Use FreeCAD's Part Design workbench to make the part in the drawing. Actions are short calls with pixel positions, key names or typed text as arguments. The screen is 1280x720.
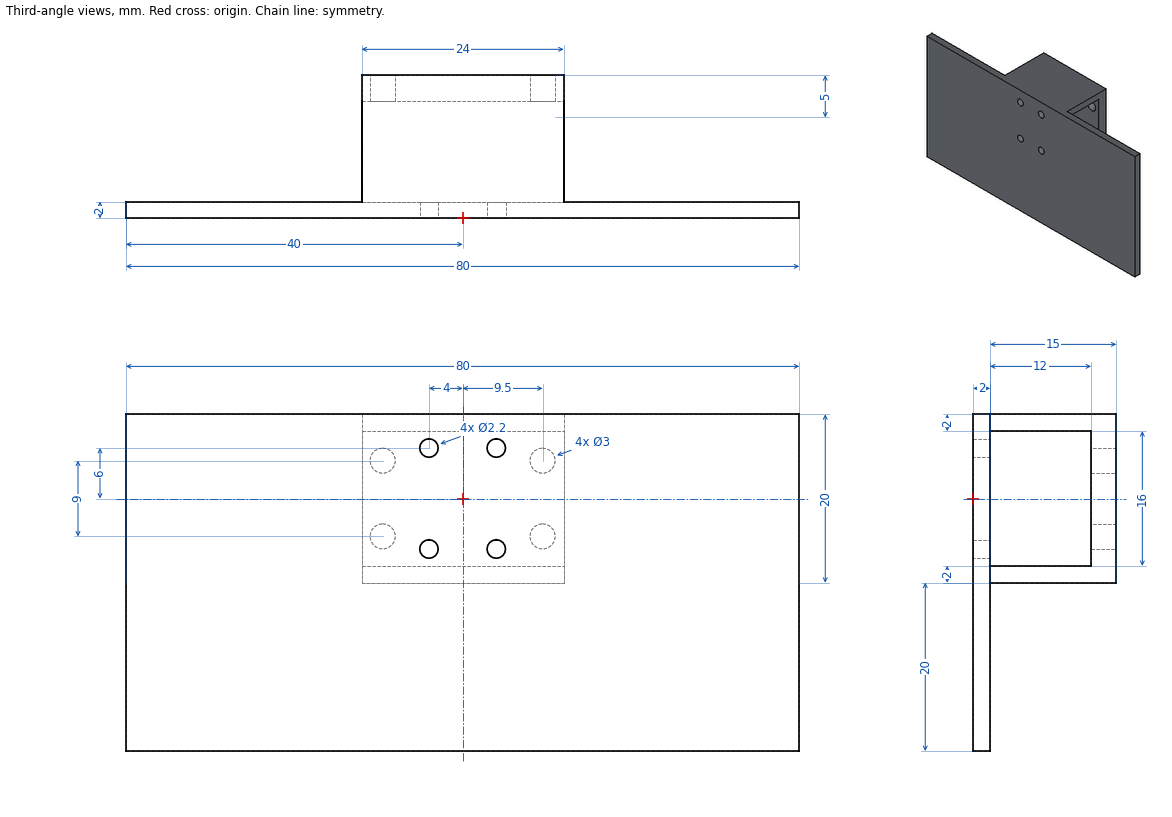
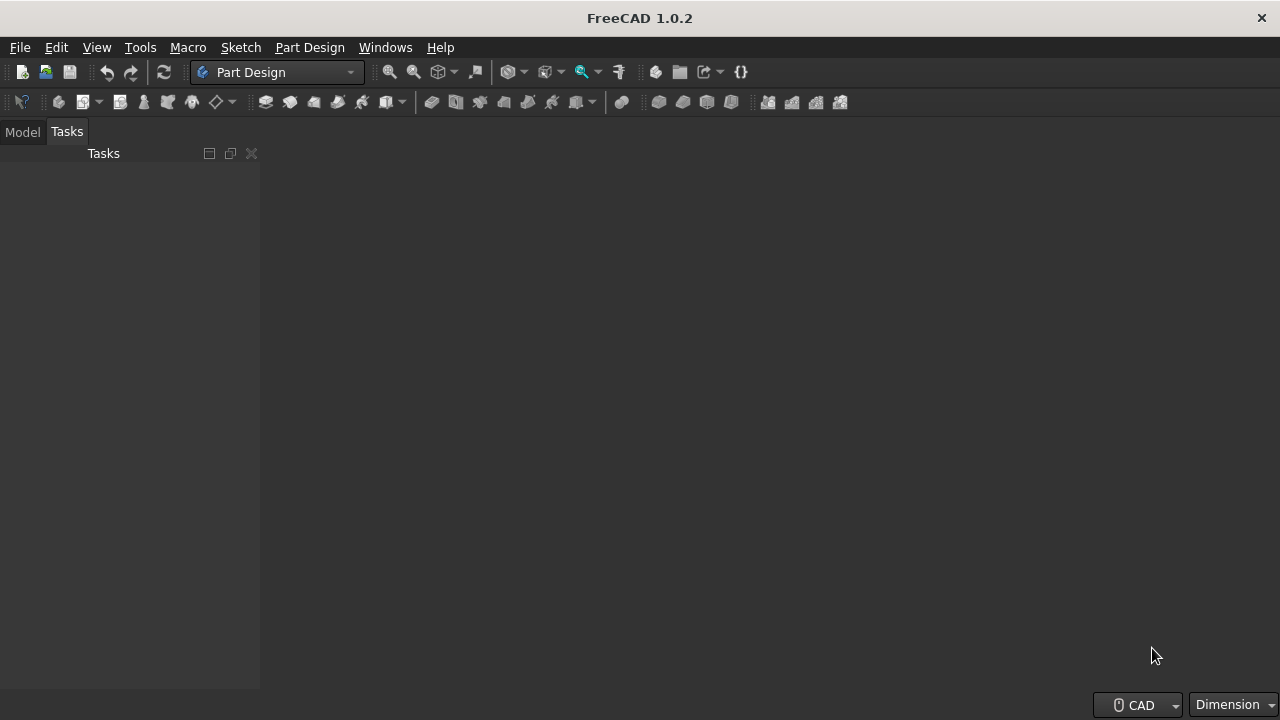
click(22, 72)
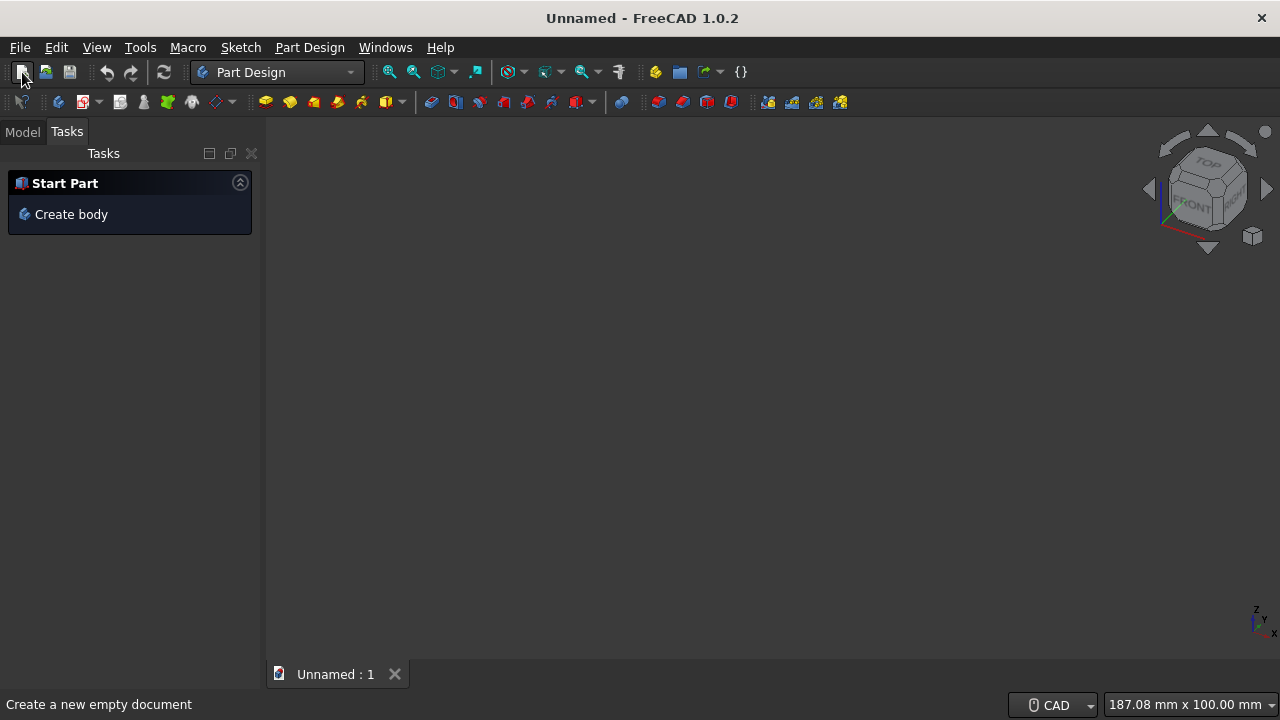
click(84, 102)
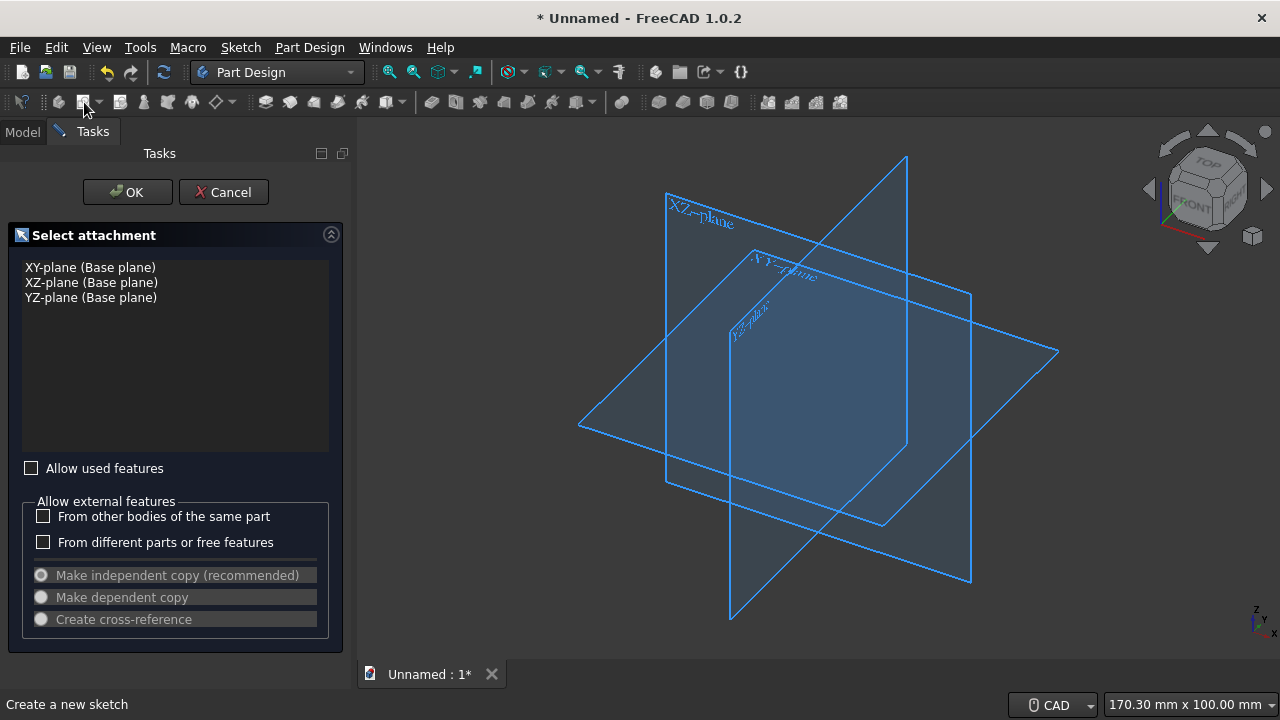
click(82, 282)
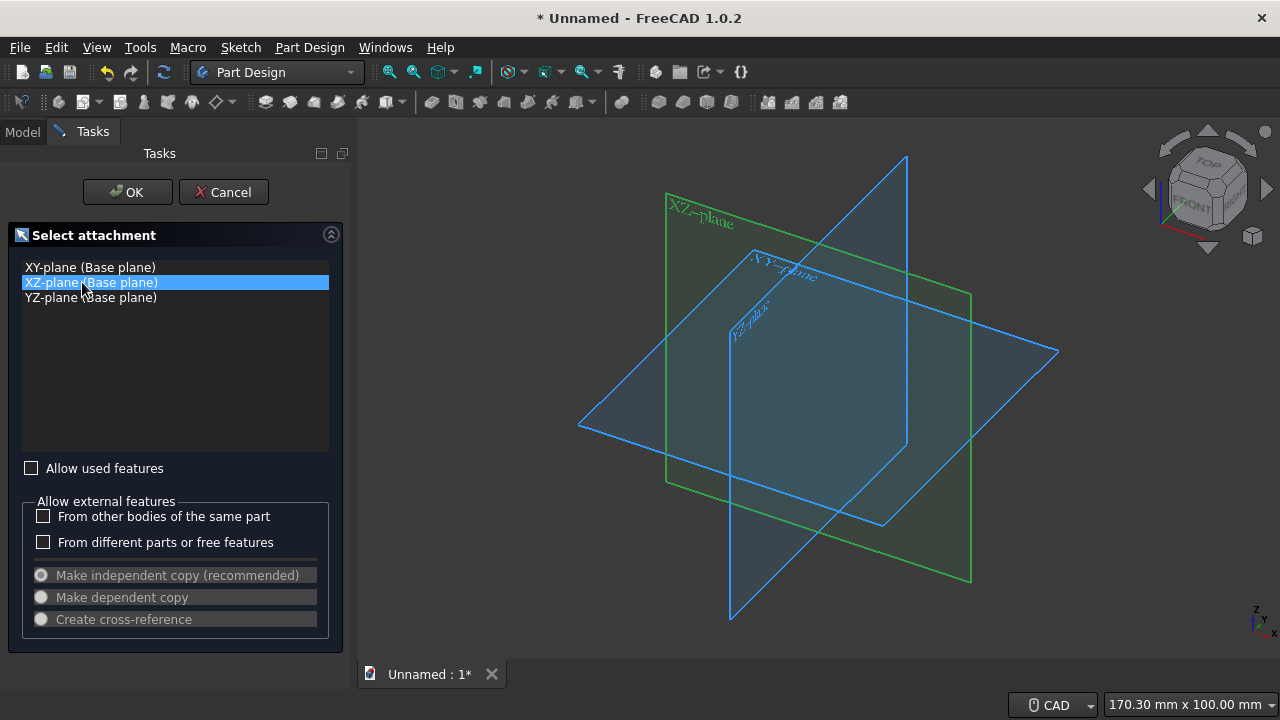
click(128, 192)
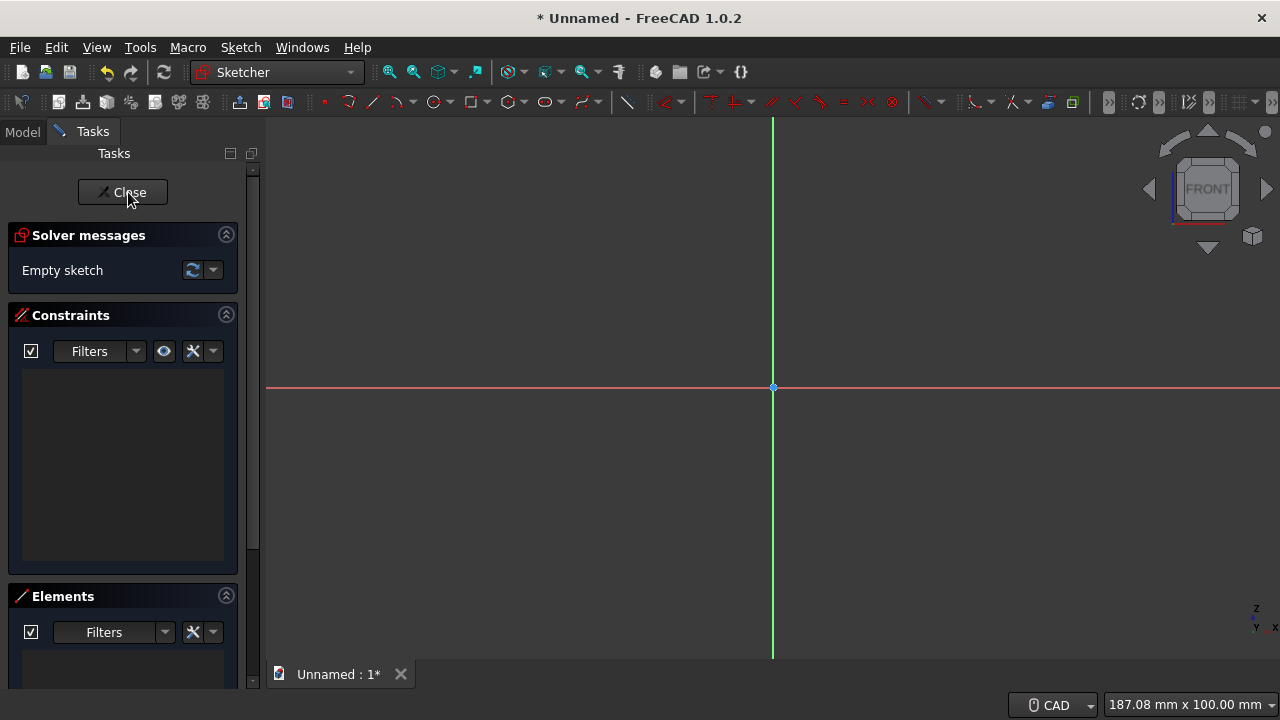
key(g)
key(v)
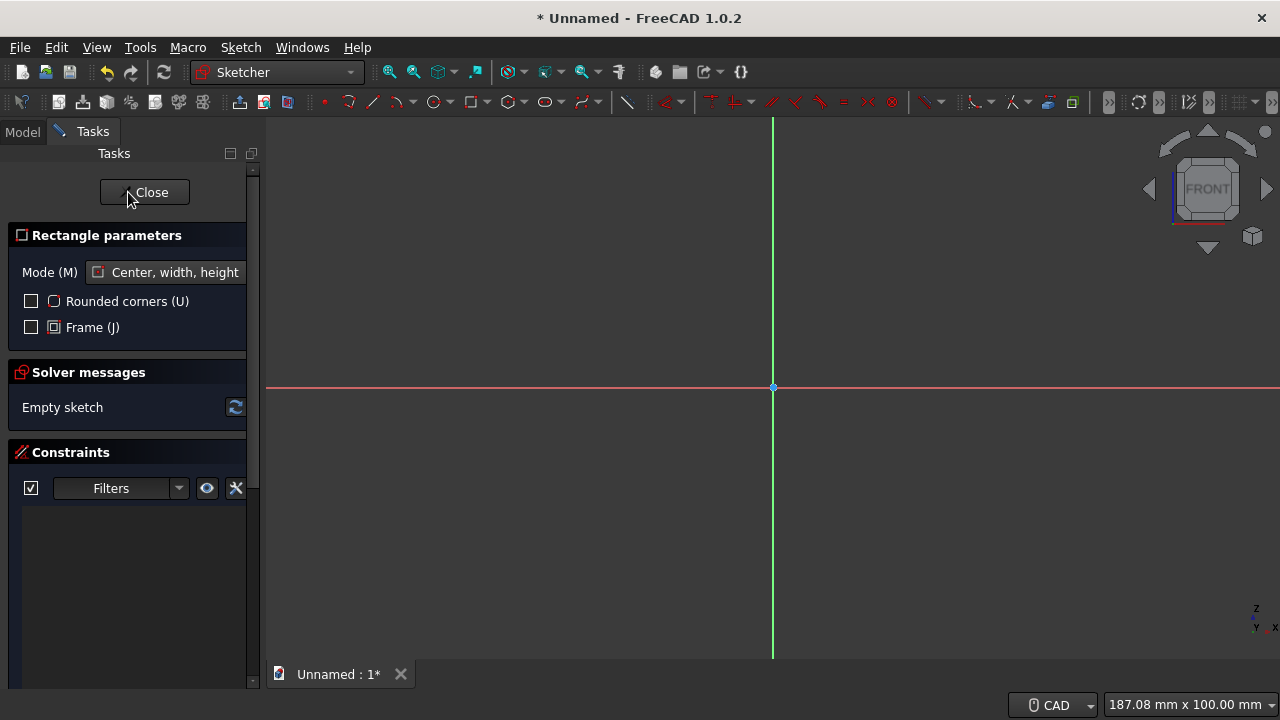
click(773, 388)
click(990, 334)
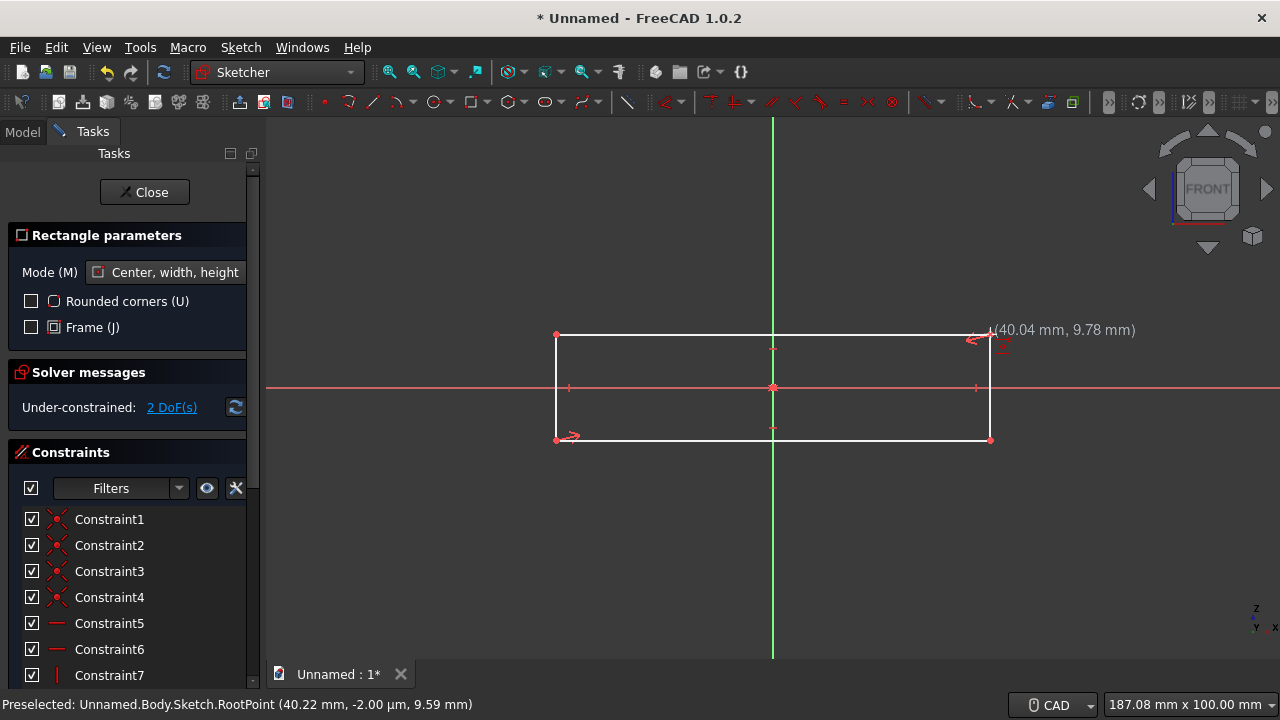
click(434, 102)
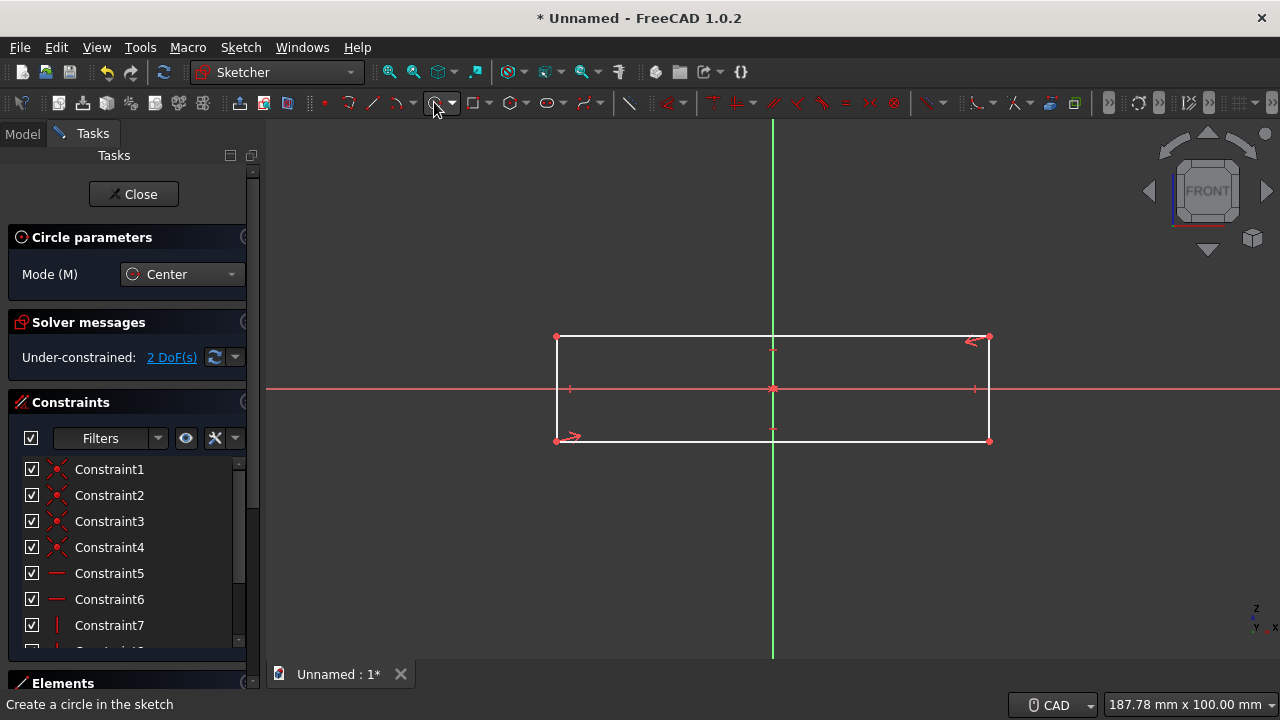
scroll(751, 357, up, 7)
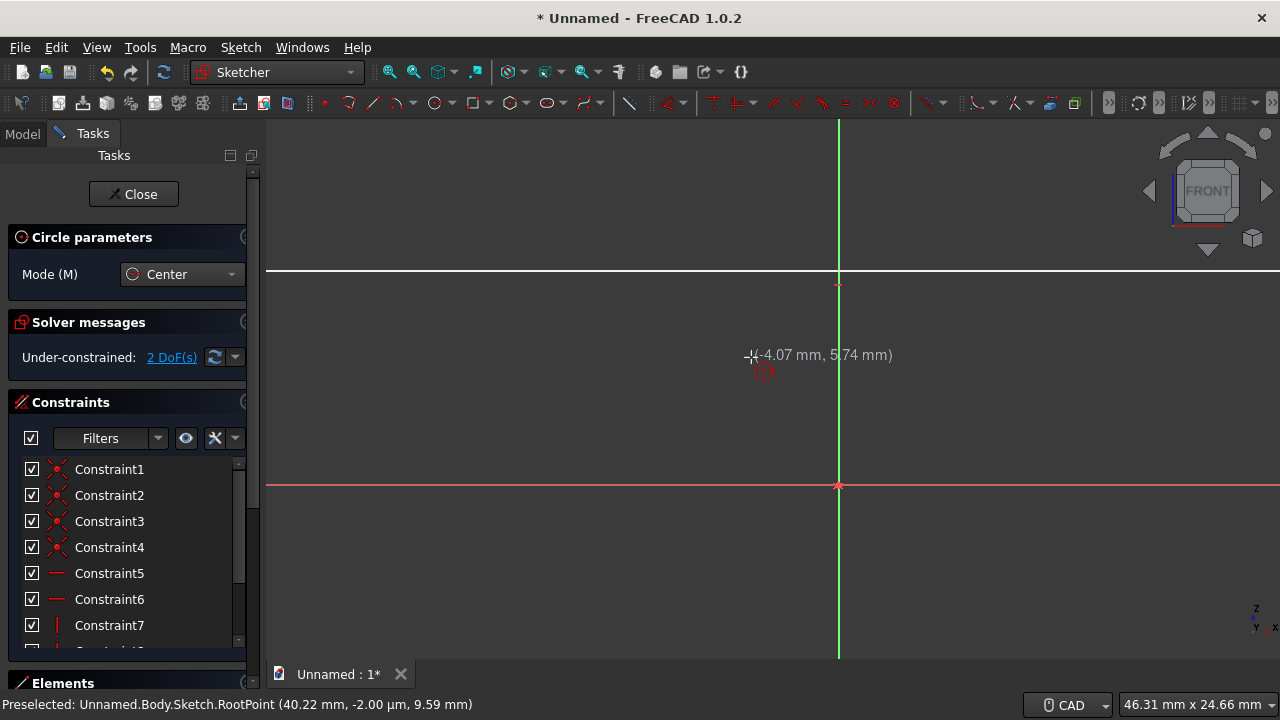
scroll(647, 347, down, 6)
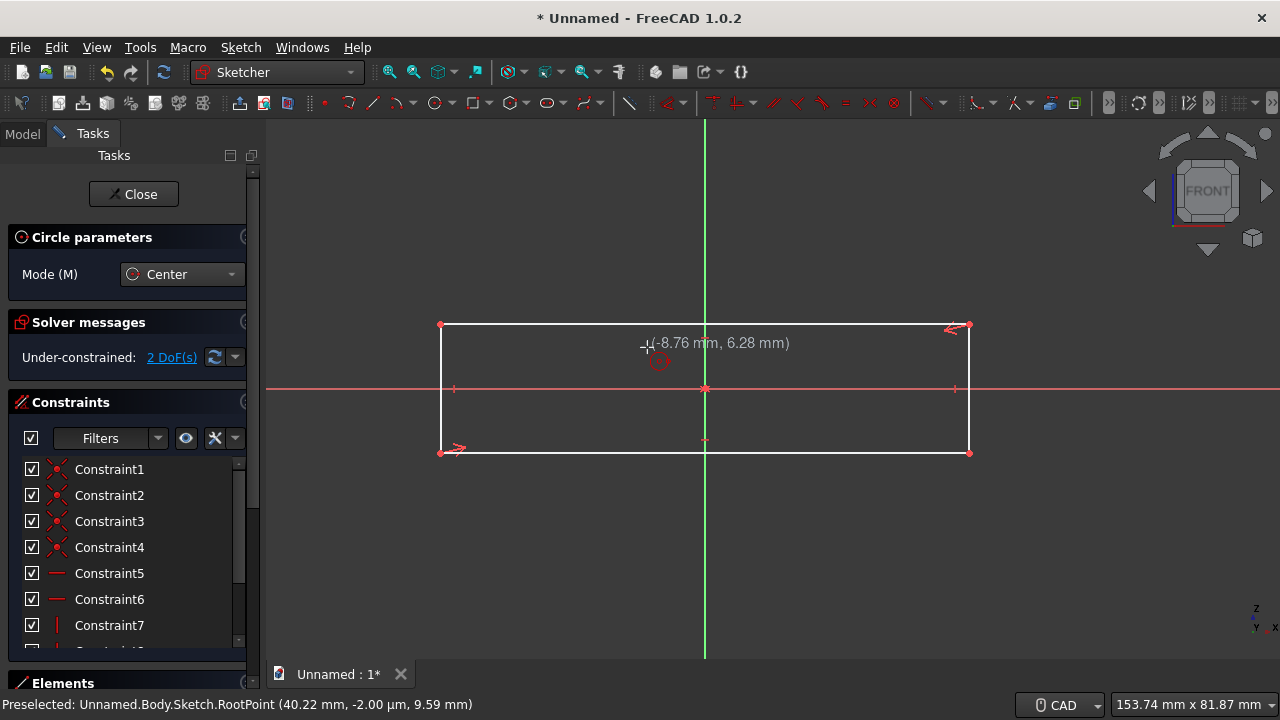
click(679, 349)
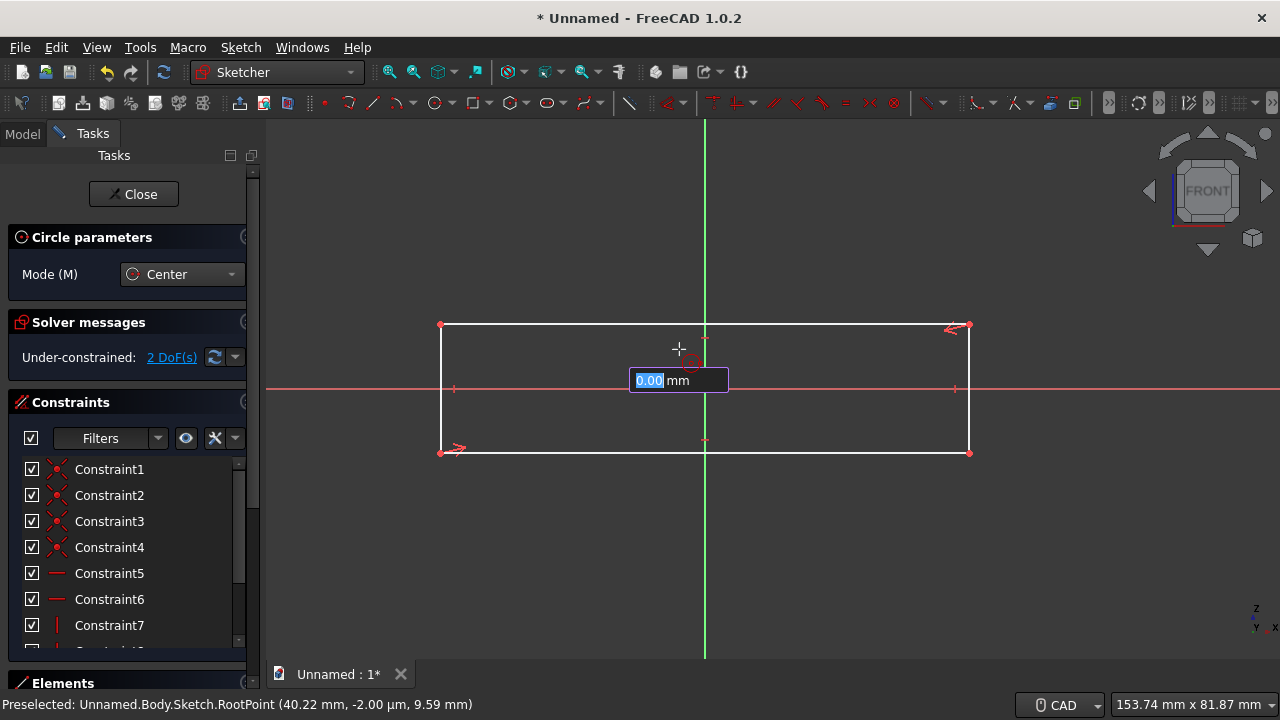
scroll(684, 344, up, 4)